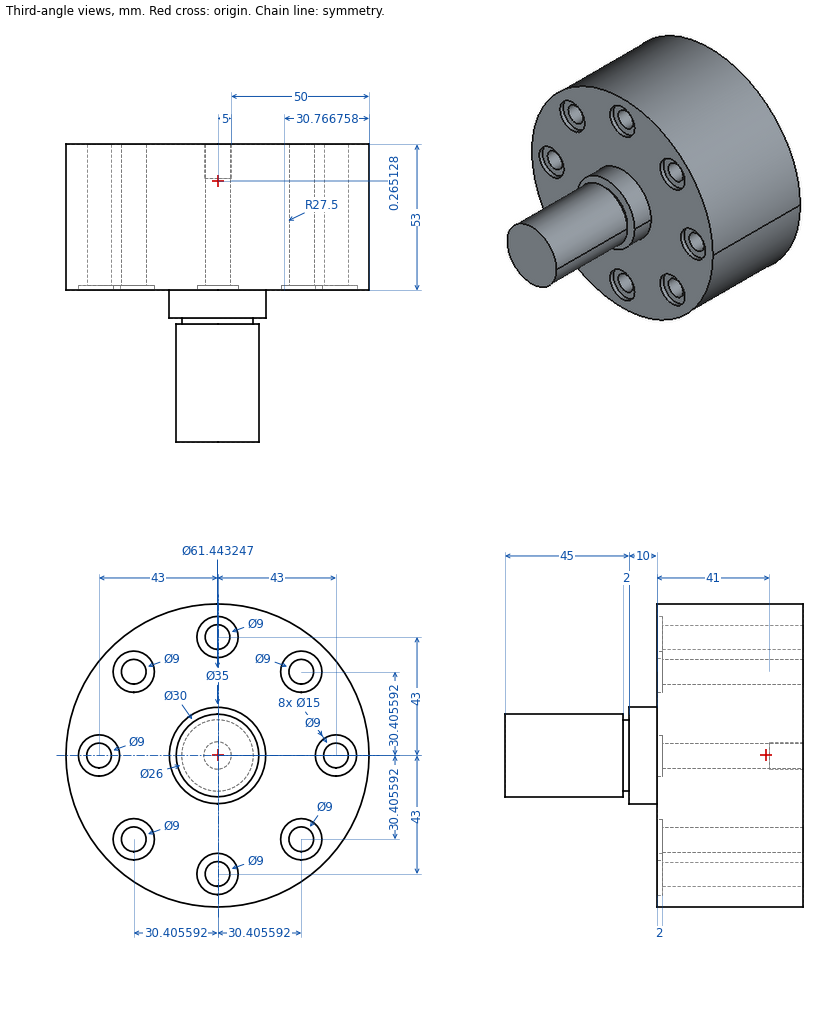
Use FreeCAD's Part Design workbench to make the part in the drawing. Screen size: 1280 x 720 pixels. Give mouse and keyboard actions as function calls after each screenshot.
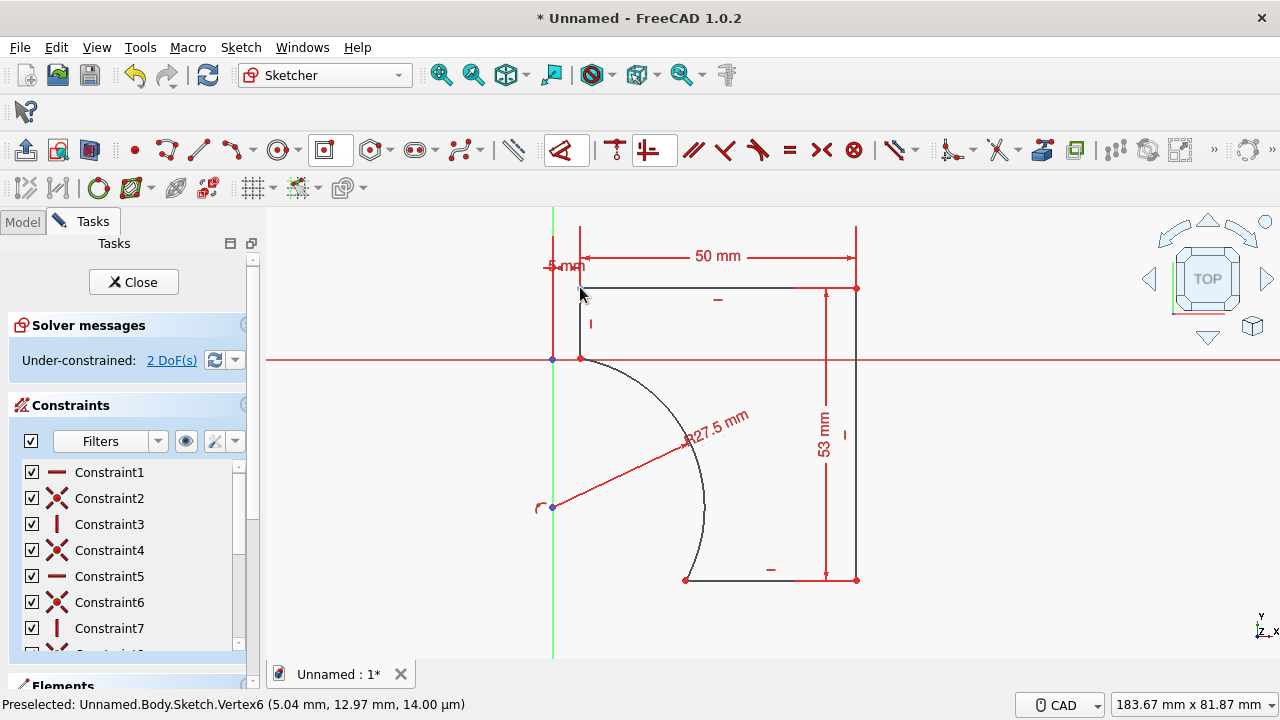
click(737, 581)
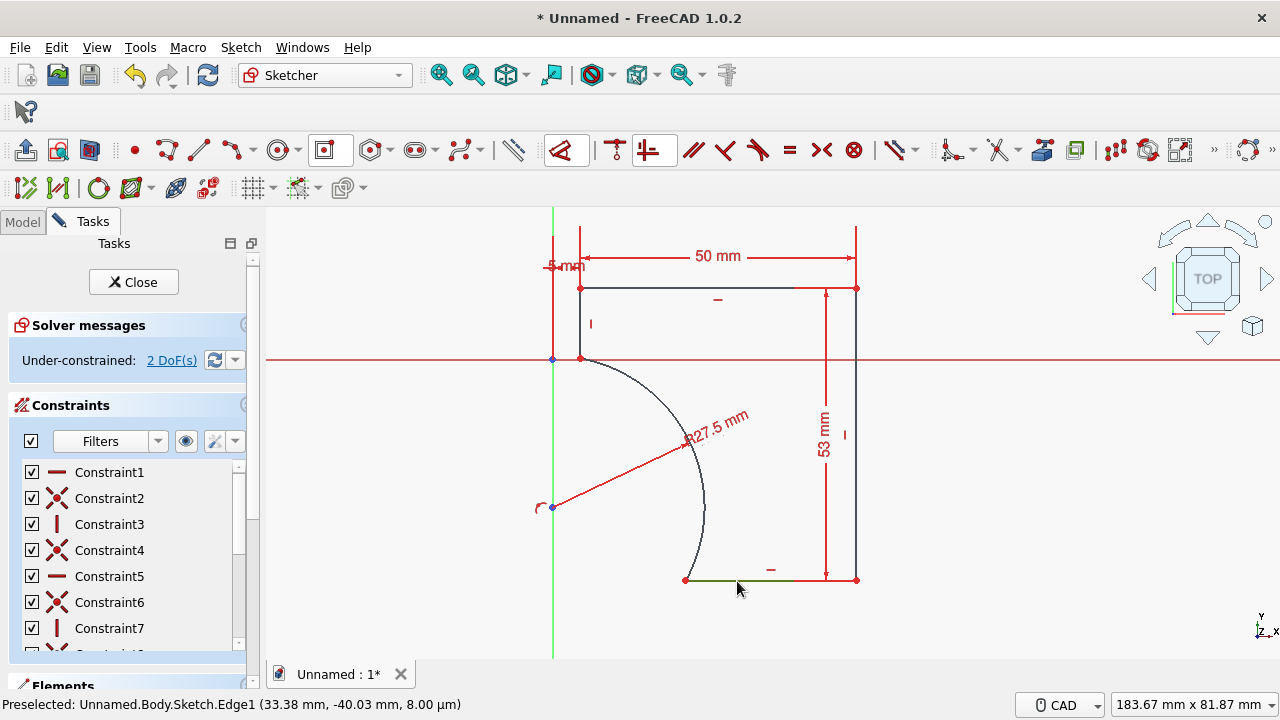
click(584, 150)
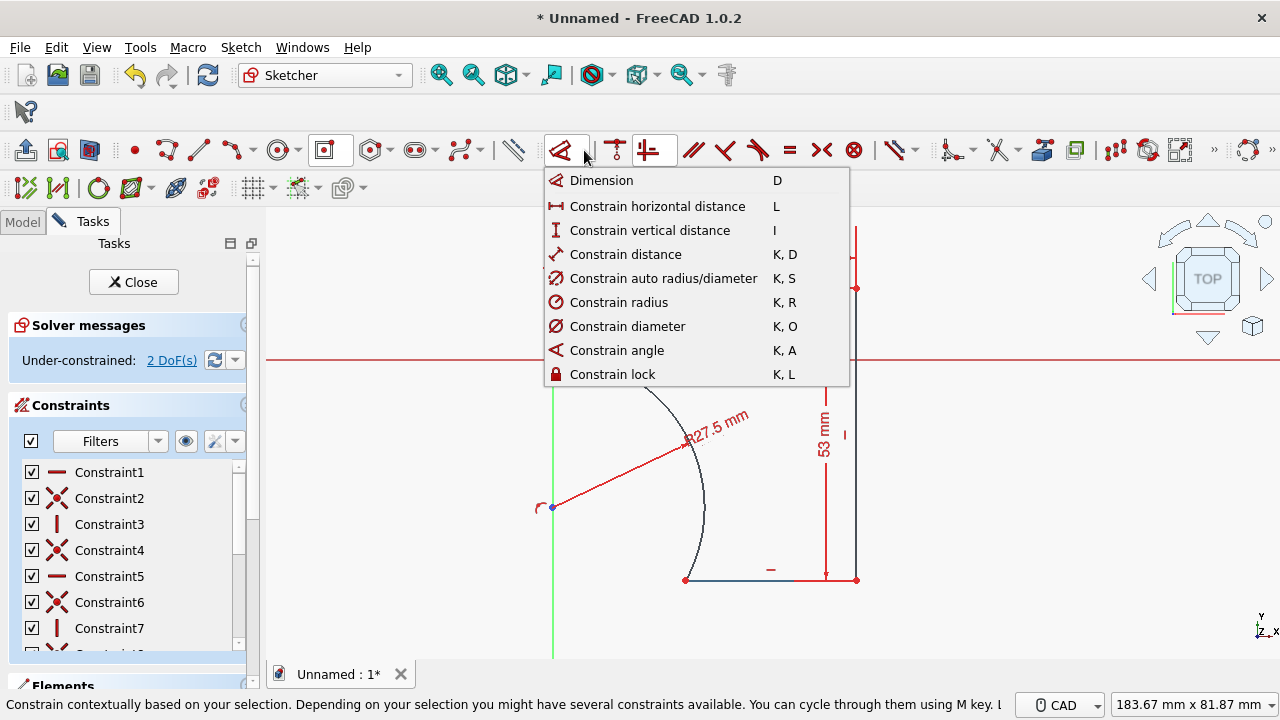
click(697, 206)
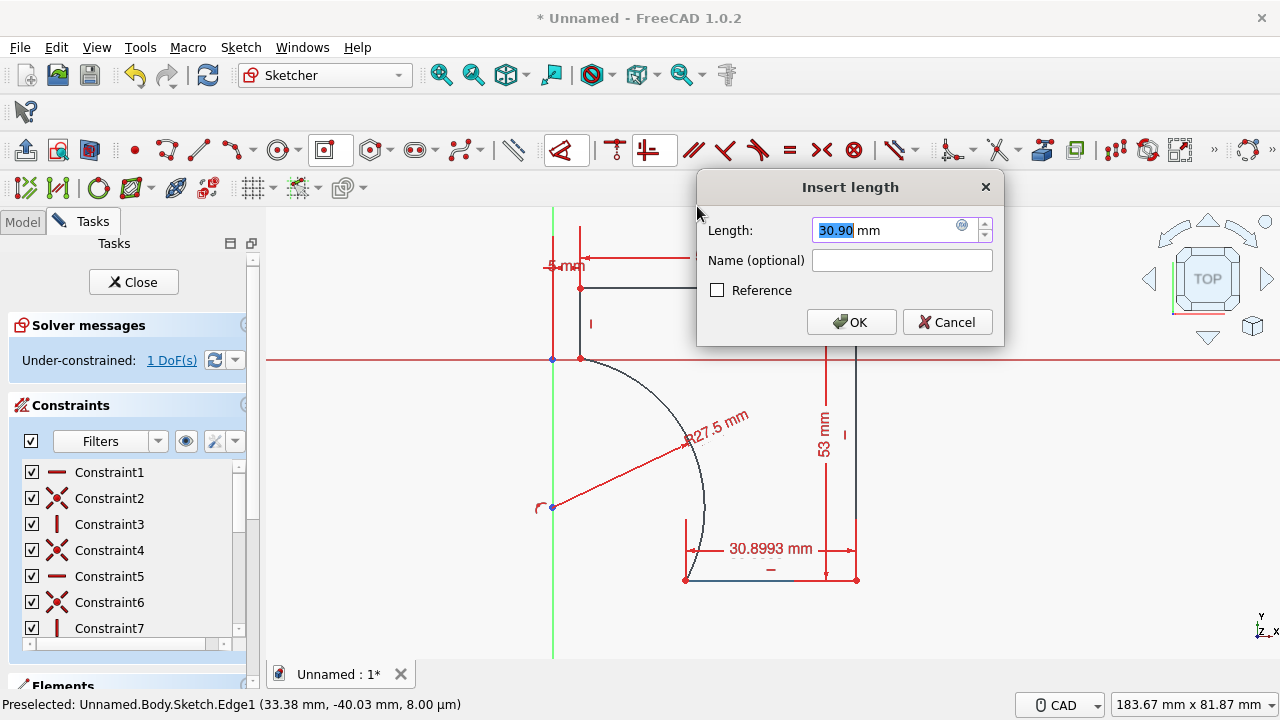
text(30.766758)
key(Return)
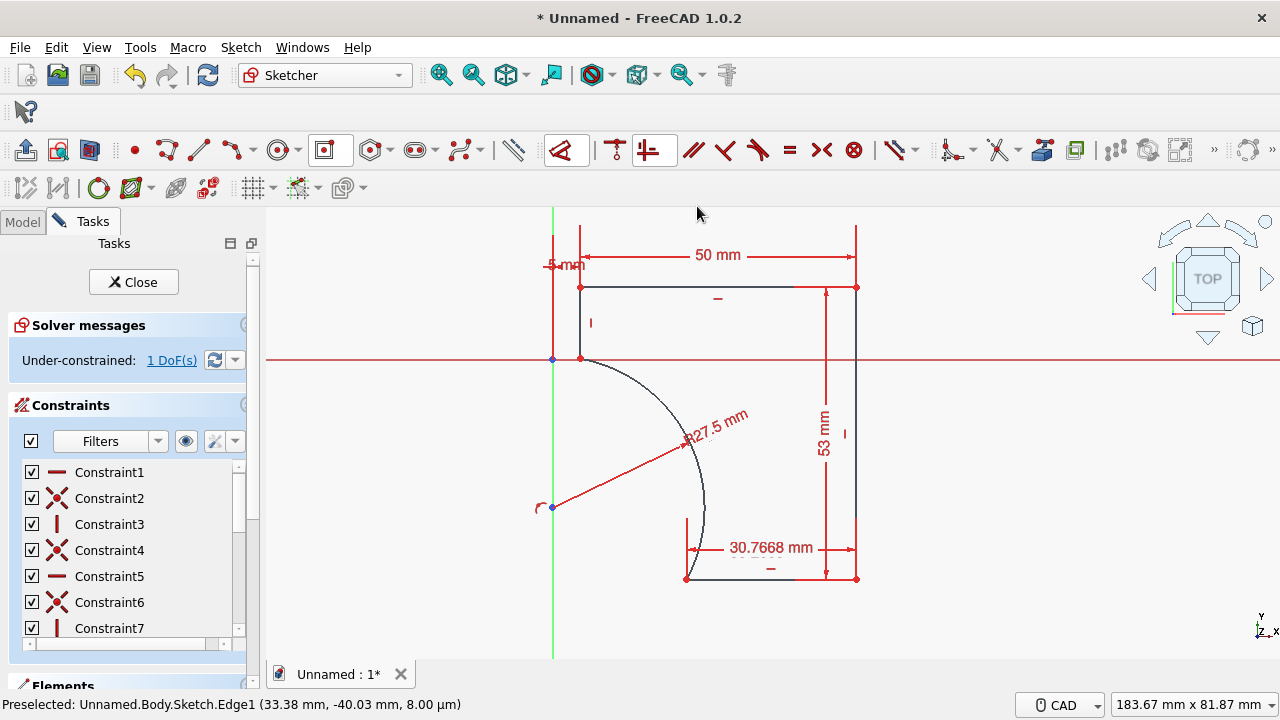
scroll(580, 359, up, 17)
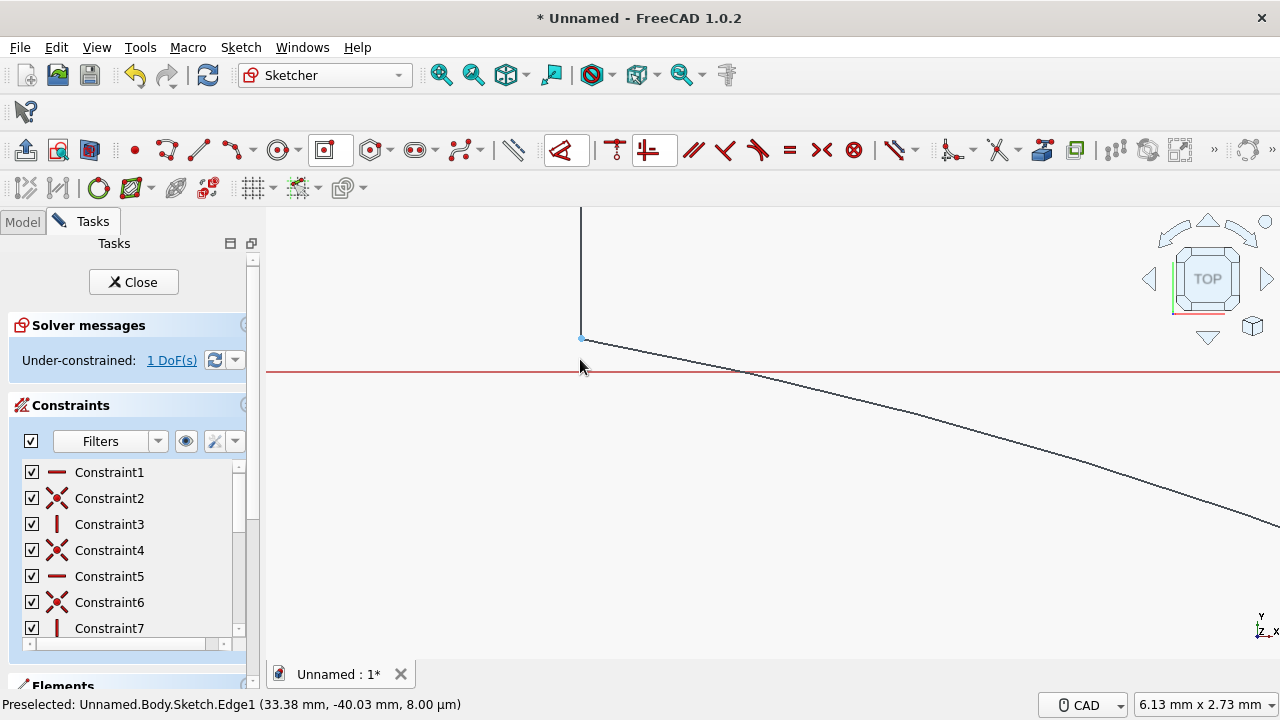
click(581, 339)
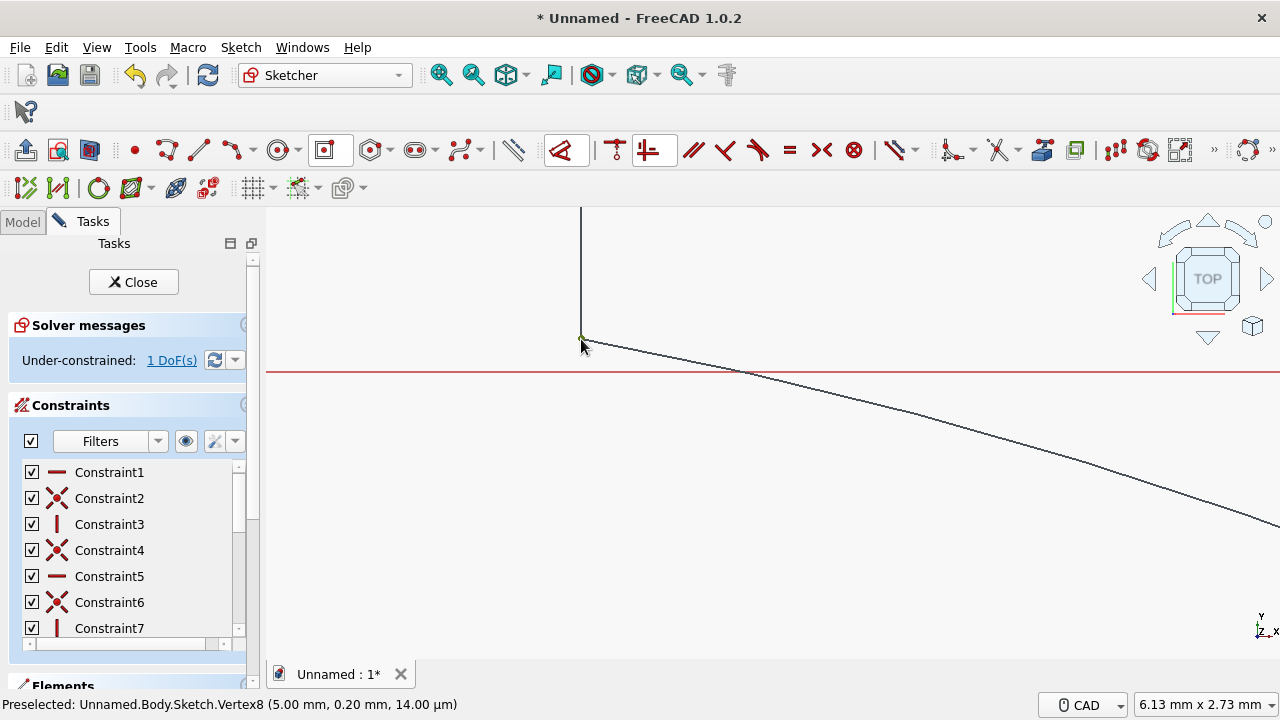
click(584, 150)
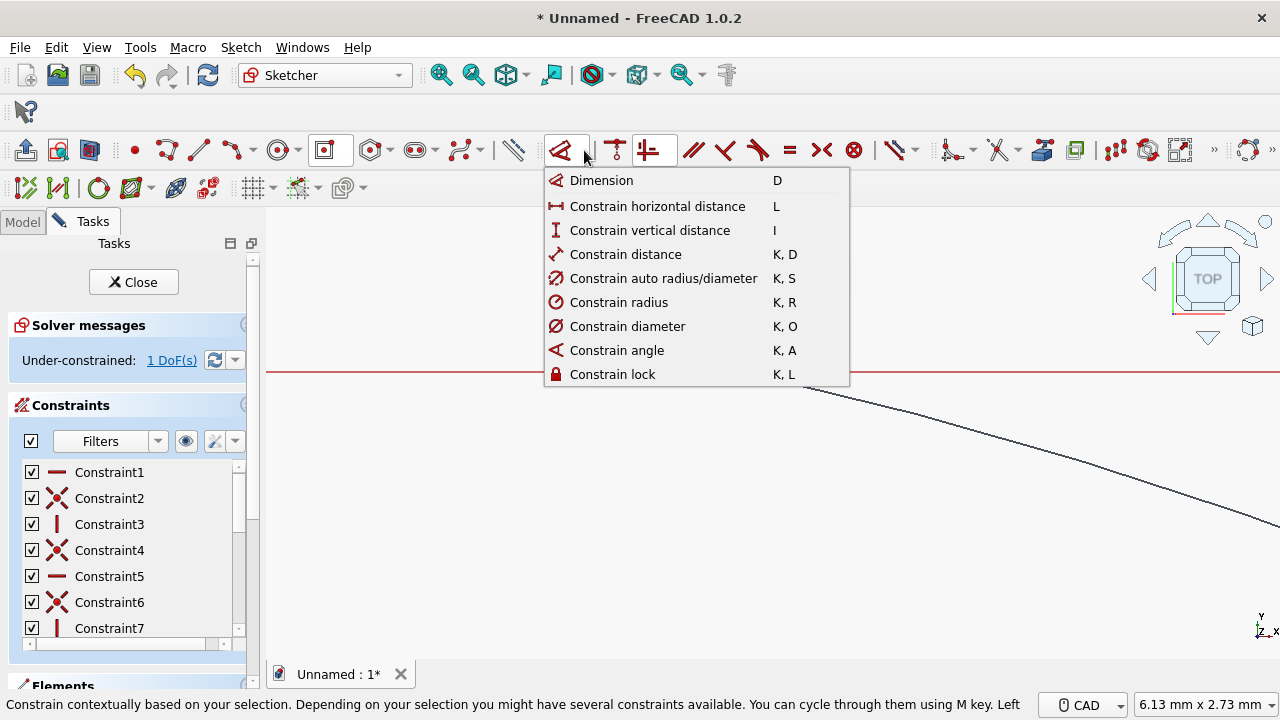
click(697, 230)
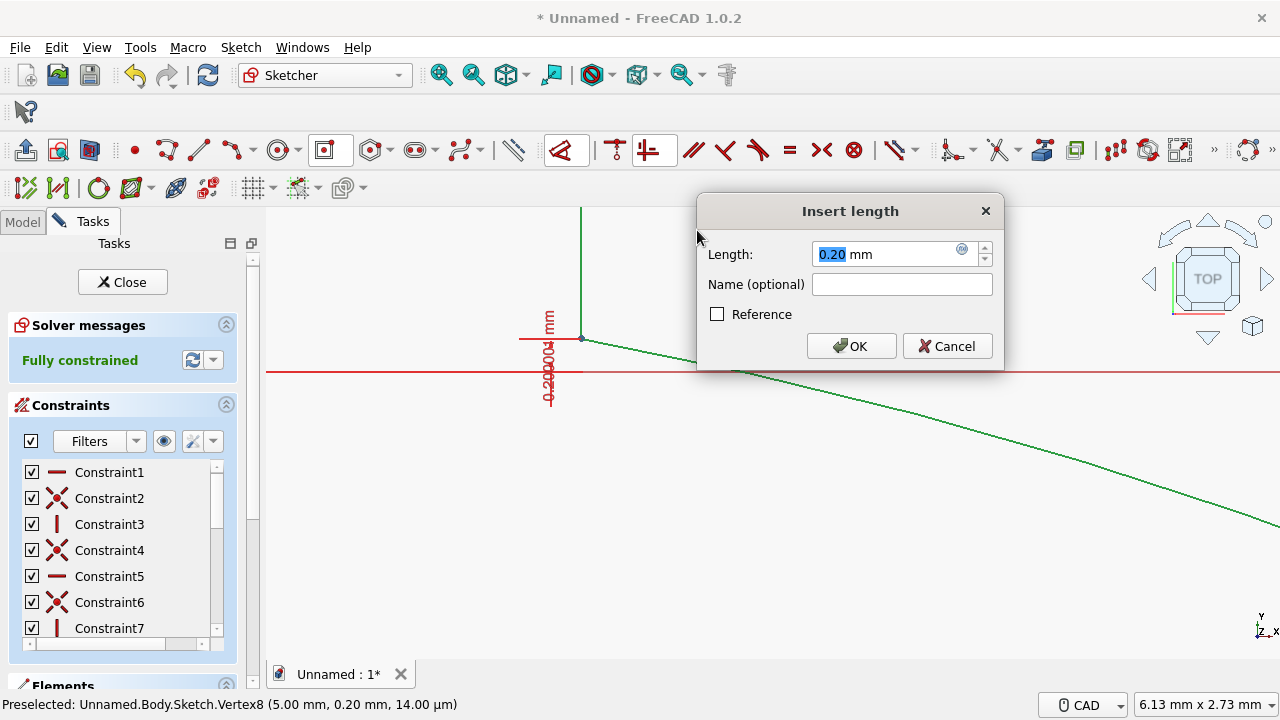
text(0.265128)
key(Return)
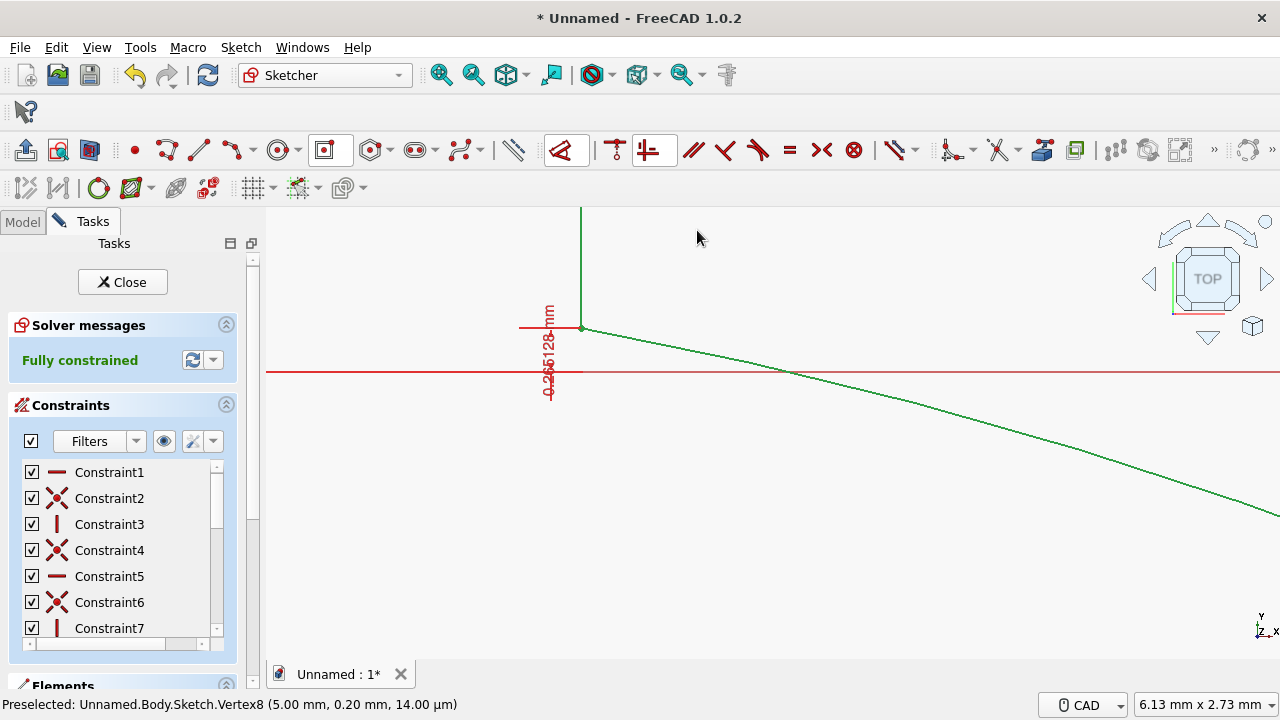
click(123, 282)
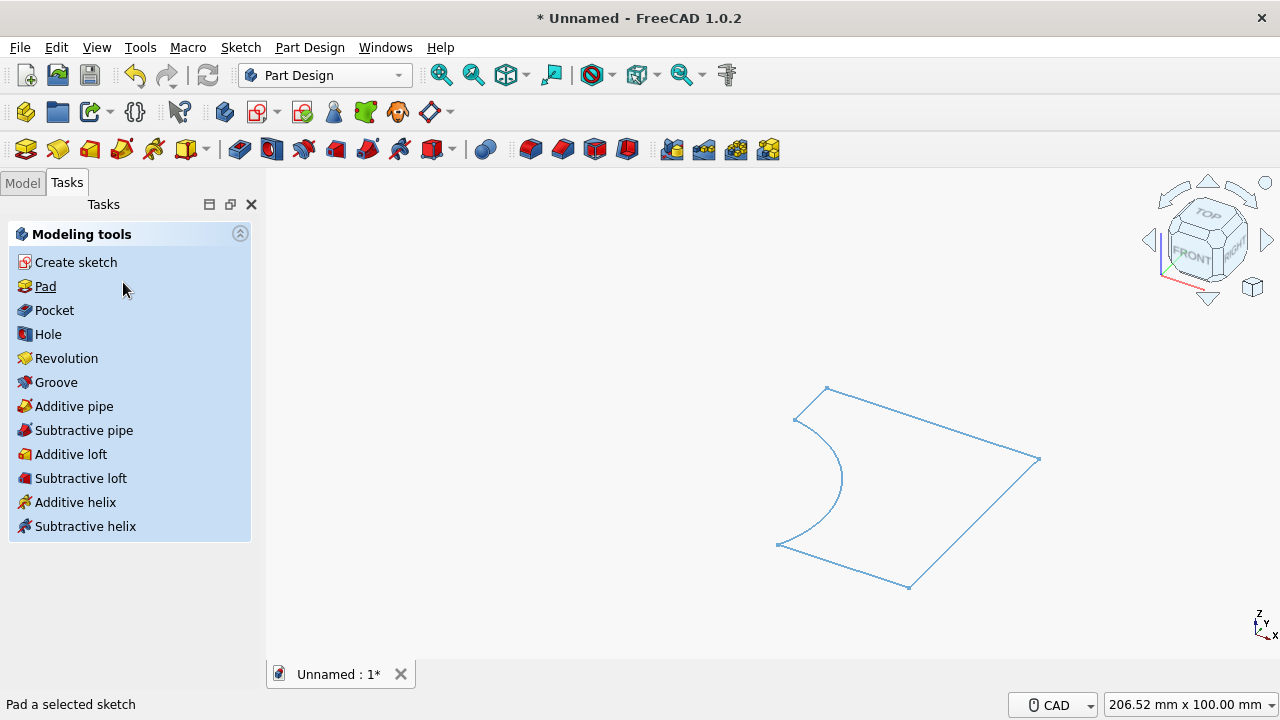
click(58, 150)